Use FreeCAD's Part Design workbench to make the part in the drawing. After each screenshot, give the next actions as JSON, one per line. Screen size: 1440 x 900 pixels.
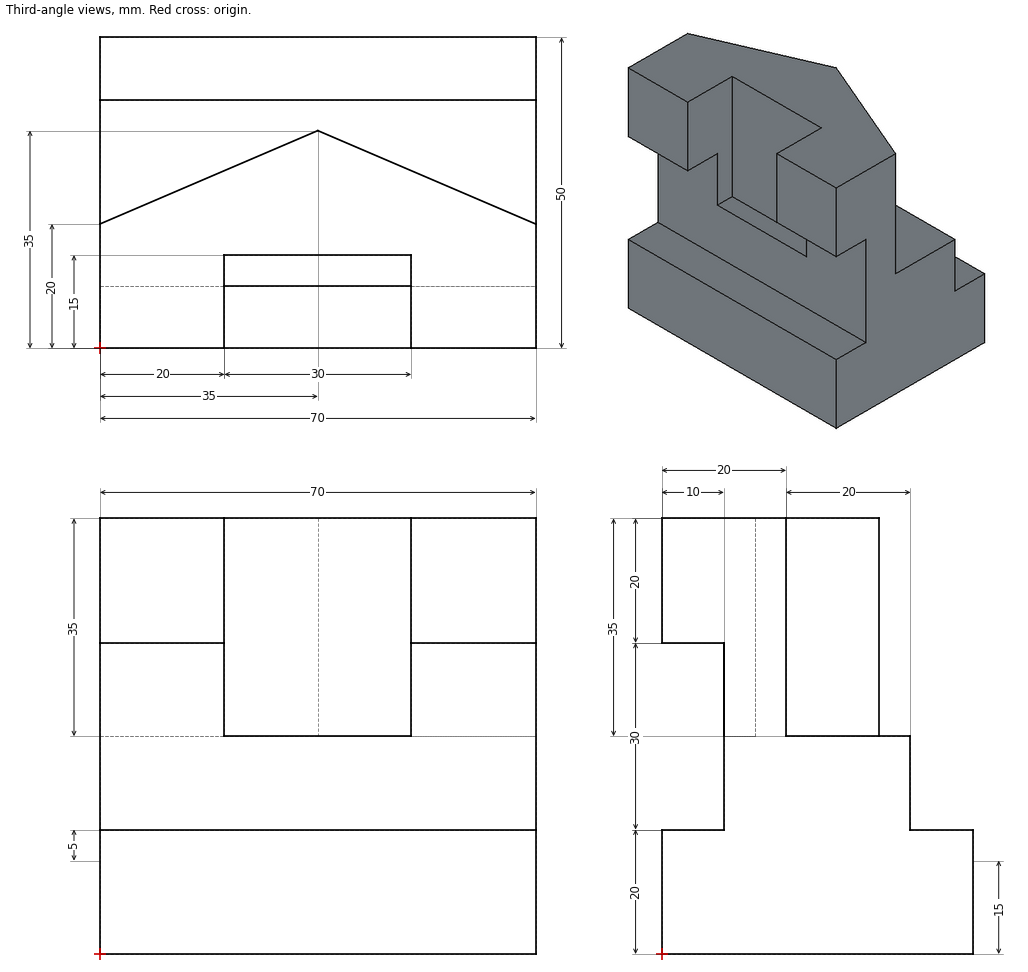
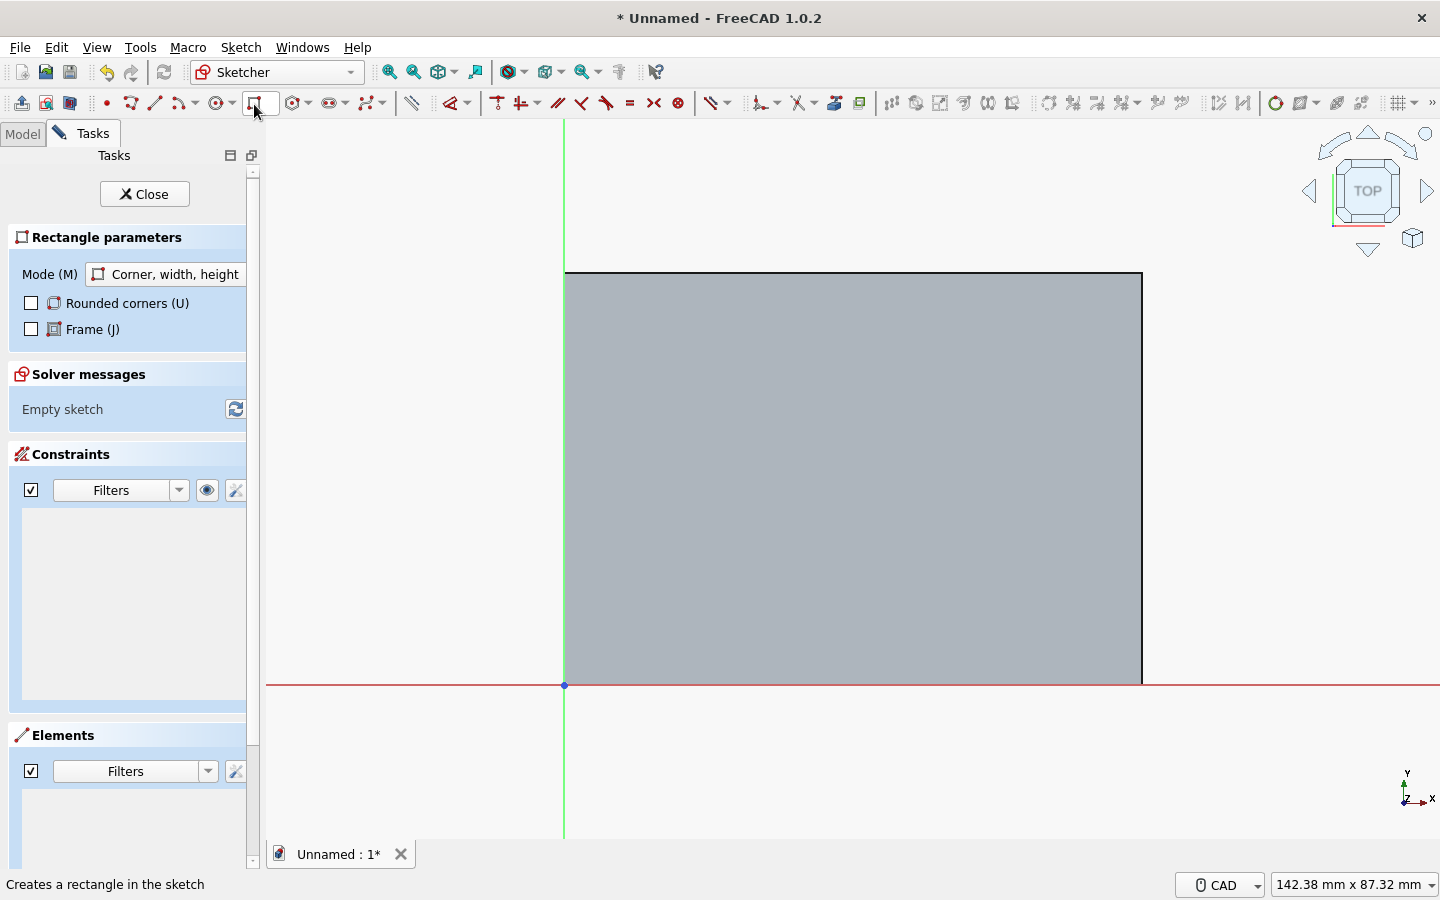
{"action": "left_click", "coordinate": [564, 685]}
{"action": "left_click", "coordinate": [1142, 273]}
{"action": "key", "text": "Escape"}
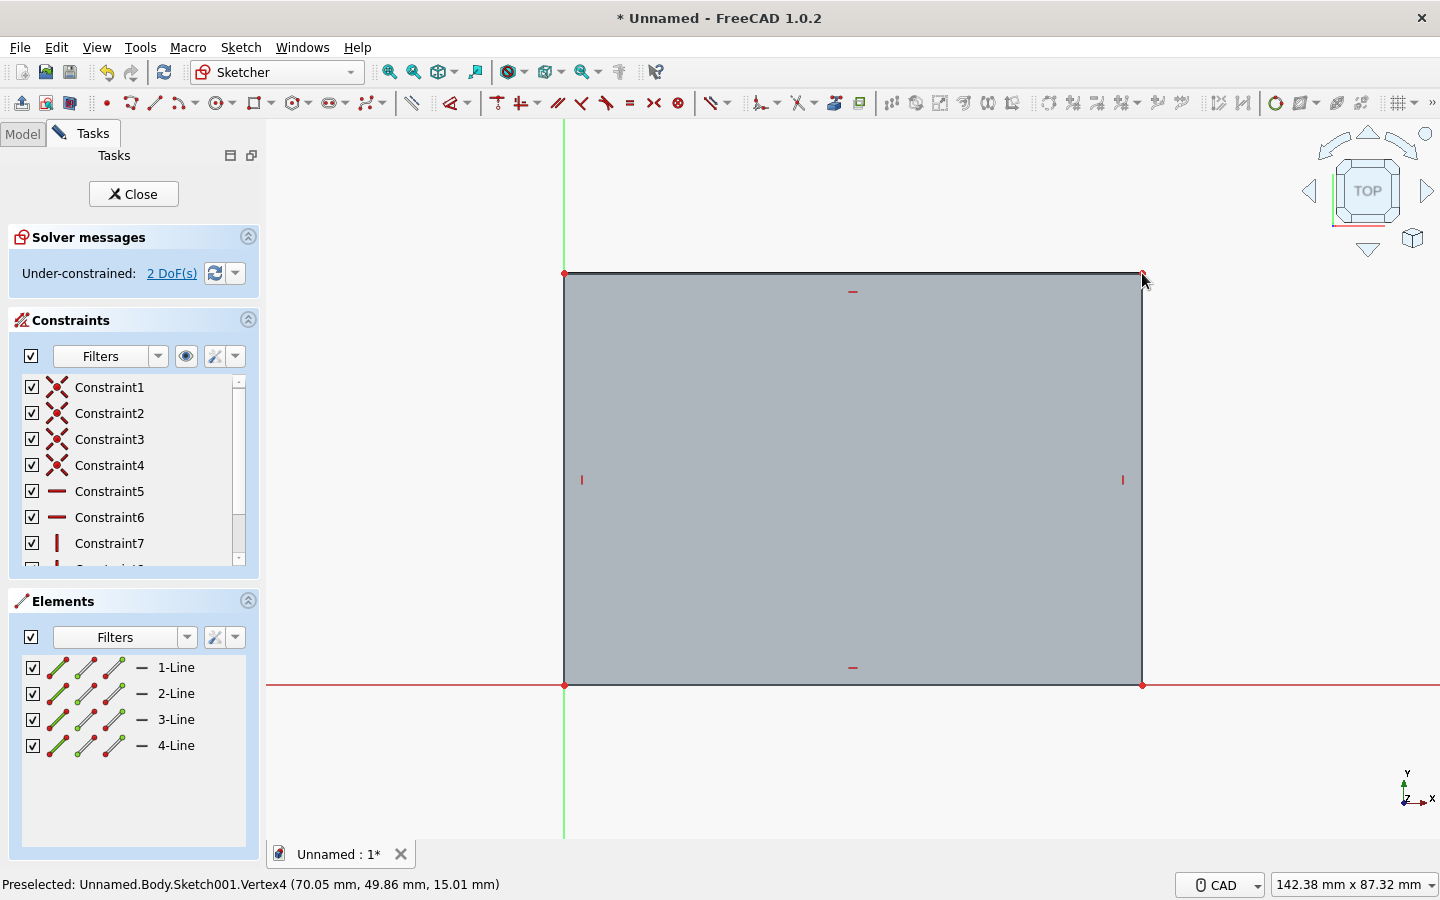
{"action": "left_click", "coordinate": [450, 104]}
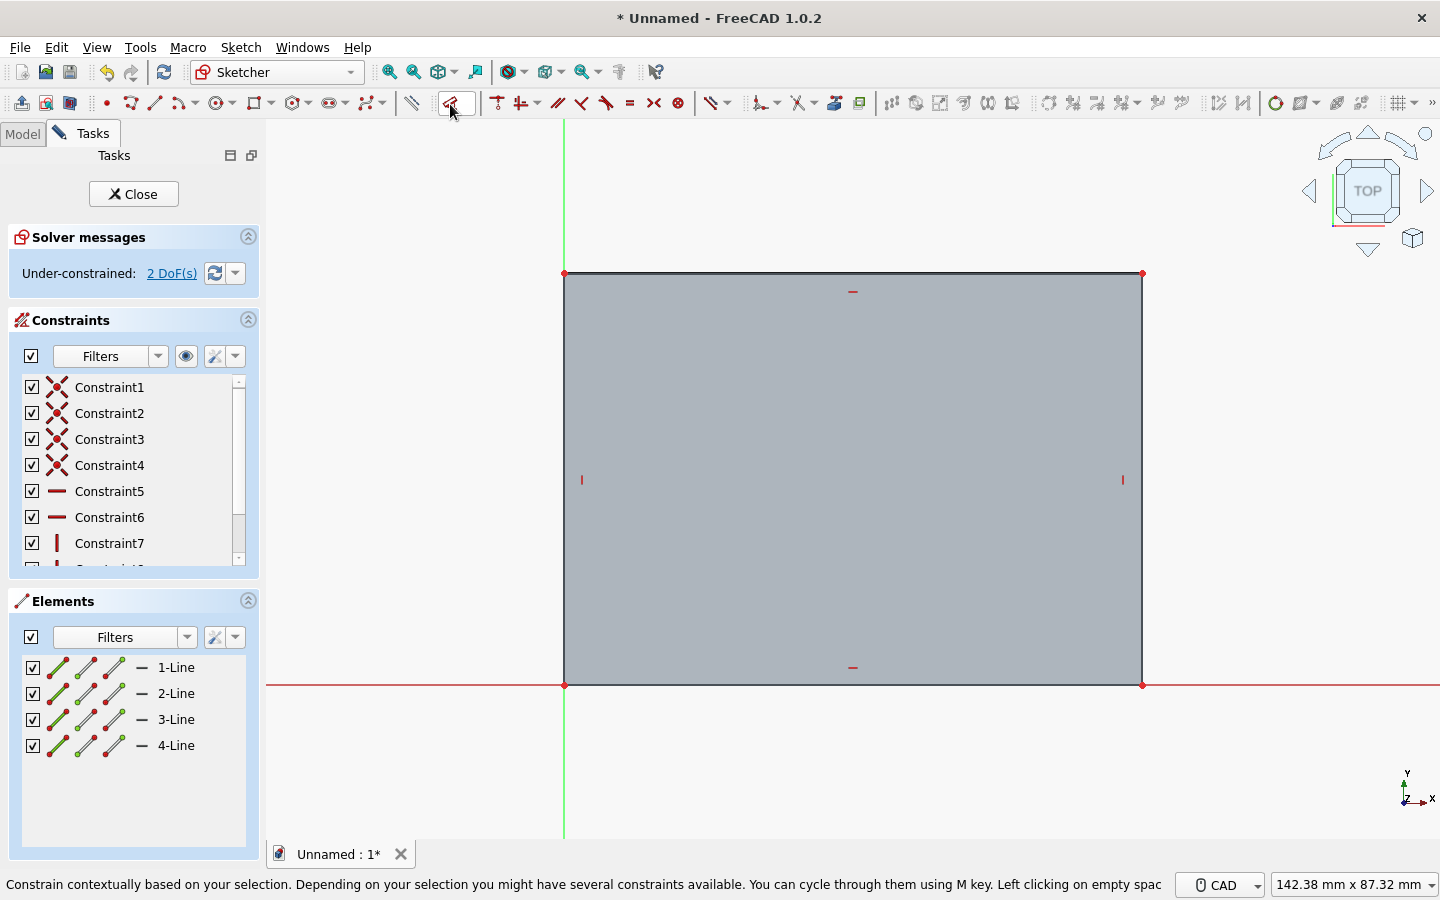
{"action": "left_click", "coordinate": [738, 685]}
{"action": "left_click", "coordinate": [853, 719]}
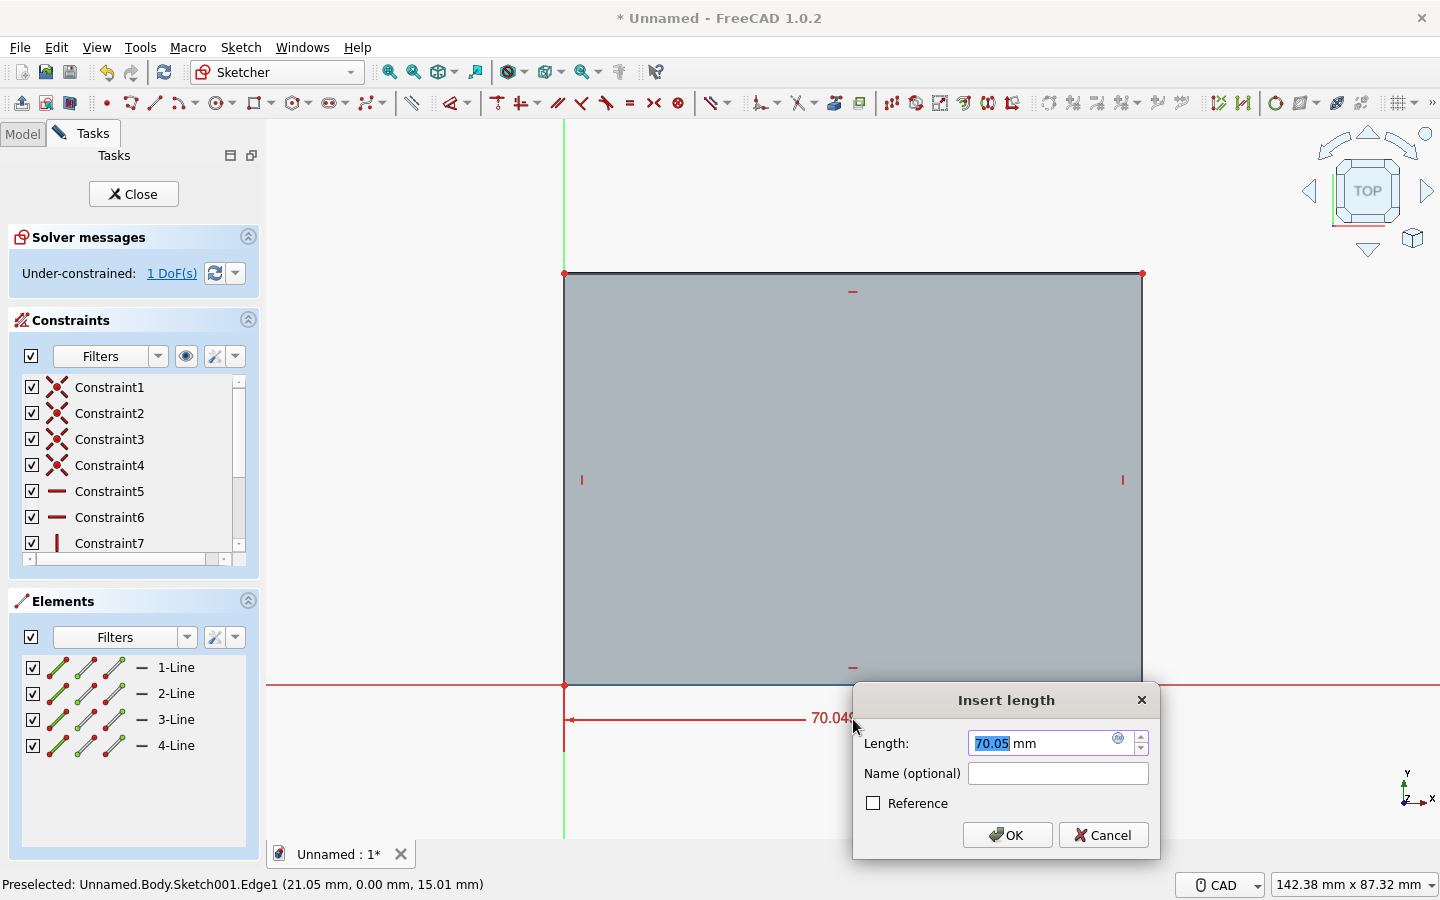
{"action": "type", "text": "70"}
{"action": "key", "text": "Return"}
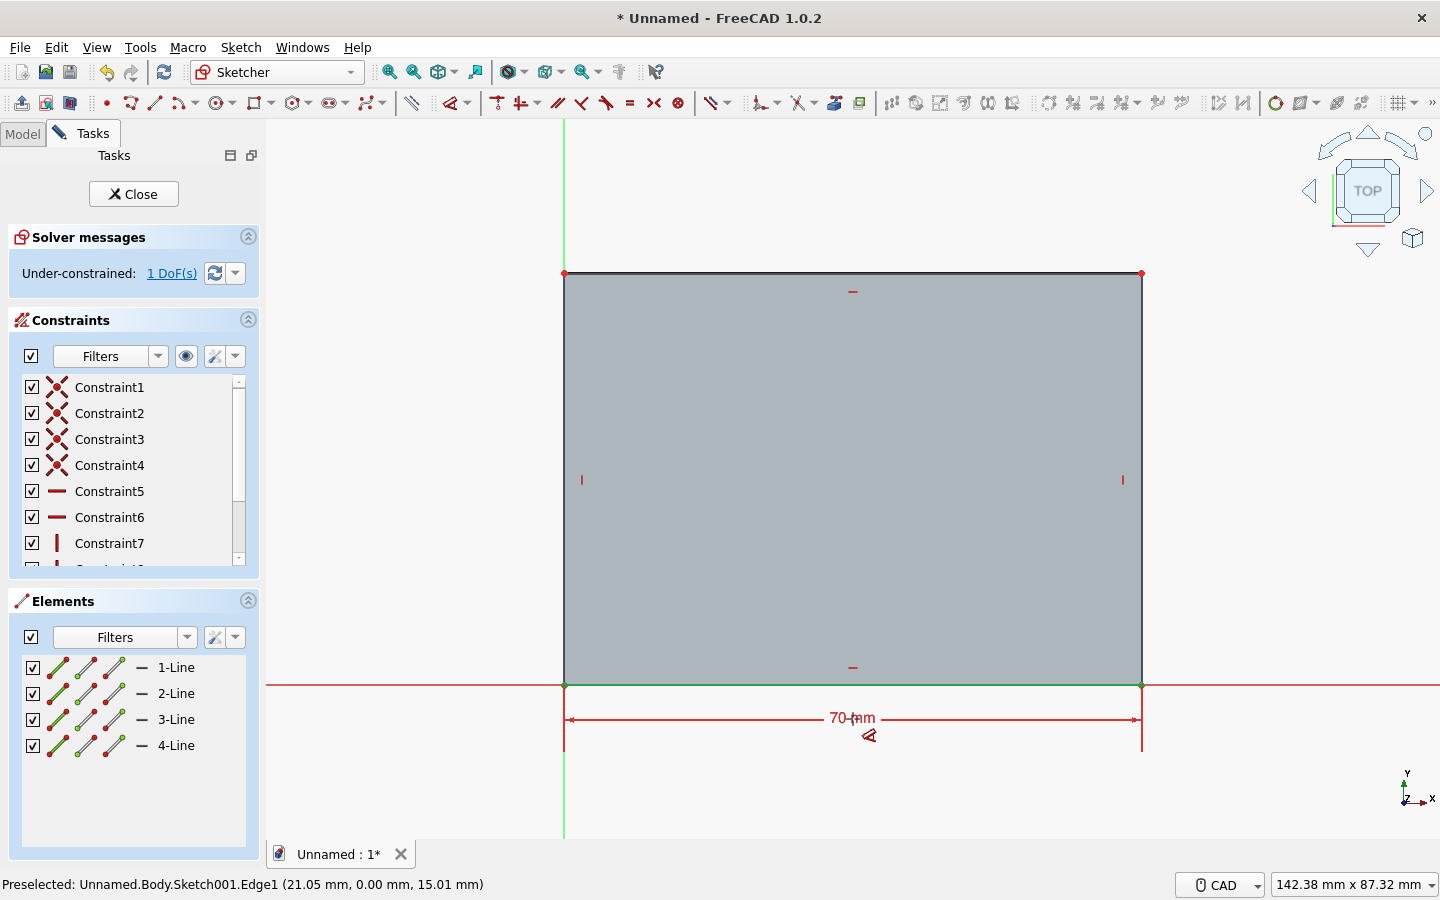
{"action": "left_click", "coordinate": [1142, 562]}
{"action": "left_click", "coordinate": [1176, 480]}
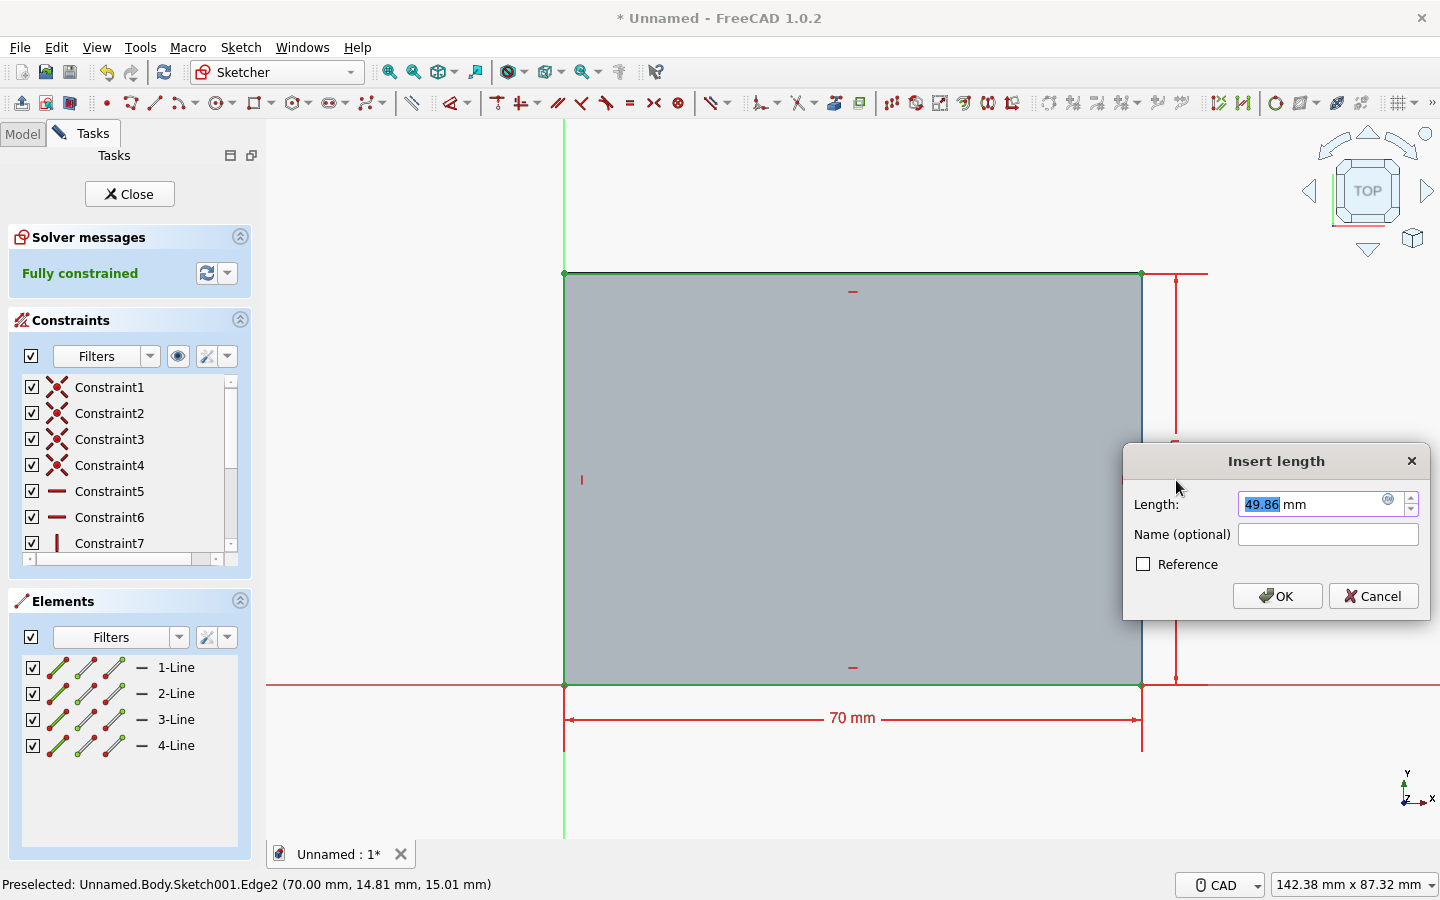
{"action": "type", "text": "50"}
{"action": "key", "text": "Return"}
{"action": "key", "text": "Escape"}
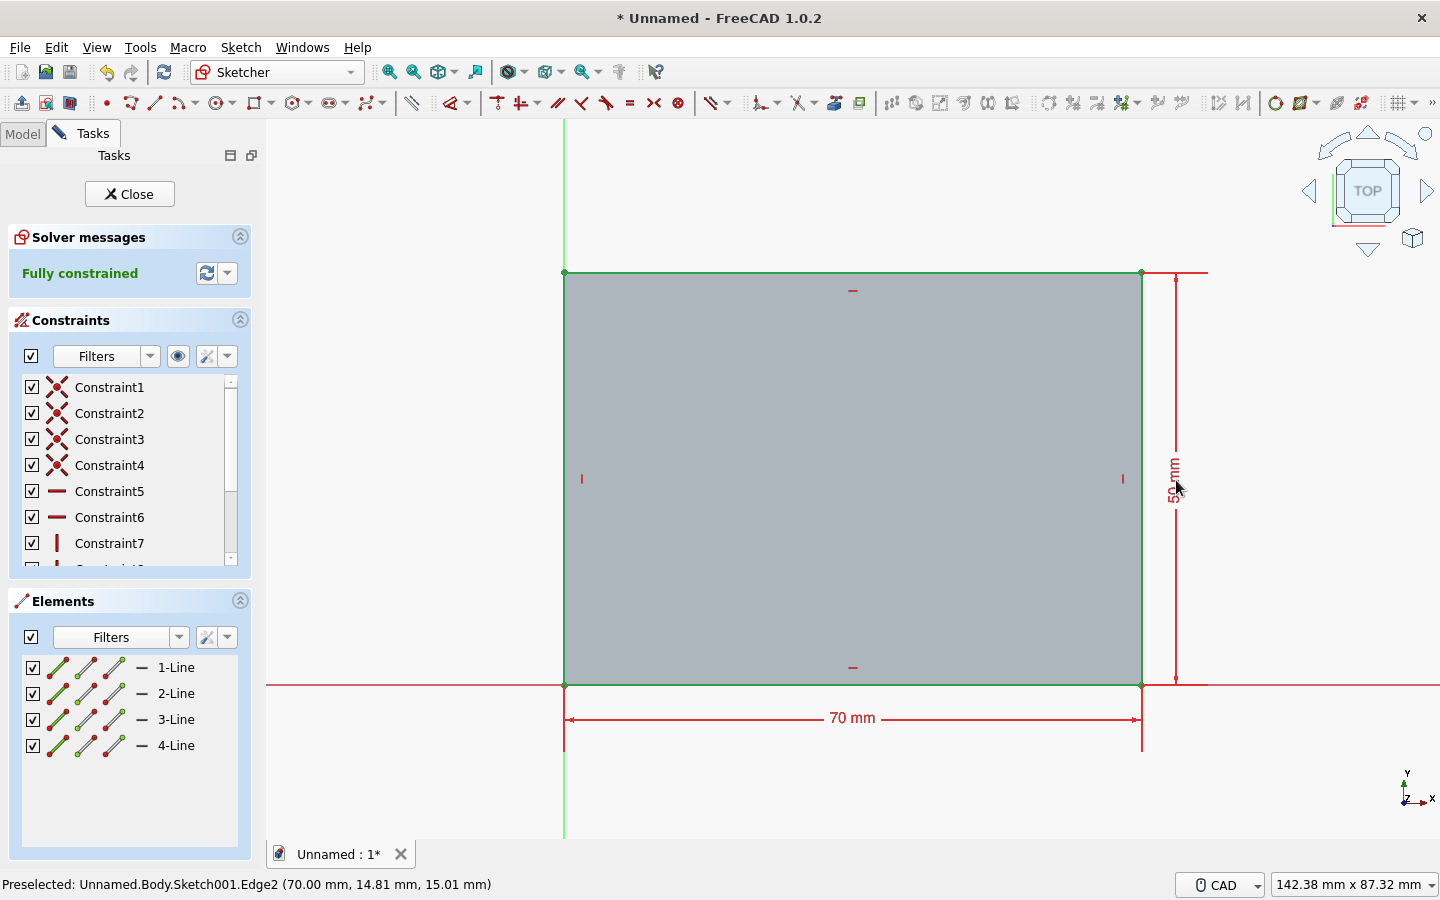
{"action": "left_click", "coordinate": [130, 194]}